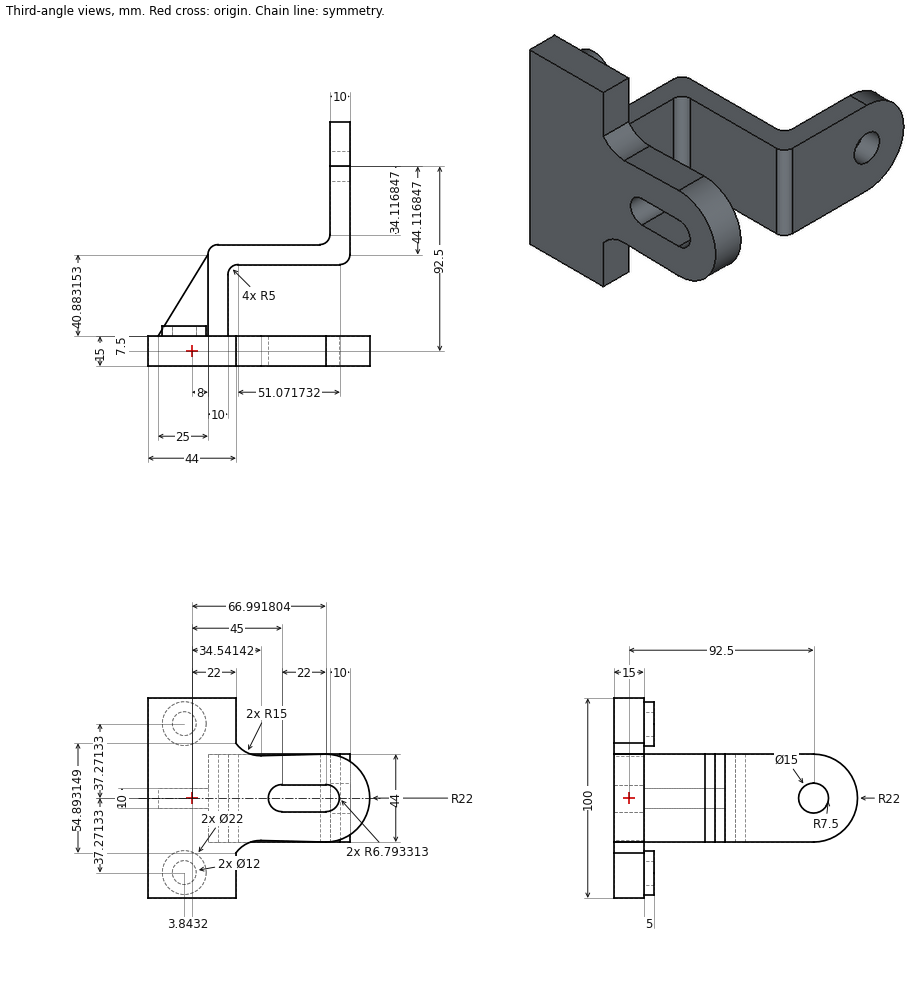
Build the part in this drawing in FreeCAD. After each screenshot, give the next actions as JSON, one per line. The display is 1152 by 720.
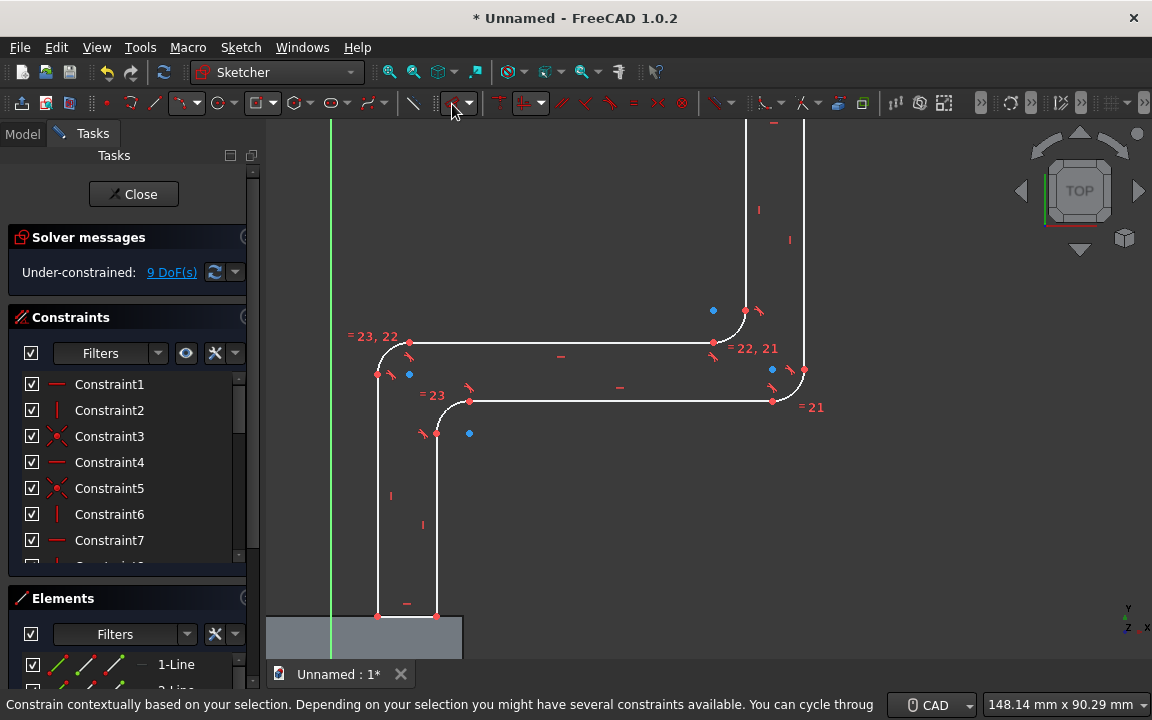
{"action": "scroll", "coordinate": [787, 398], "scroll_direction": "up", "scroll_amount": 2}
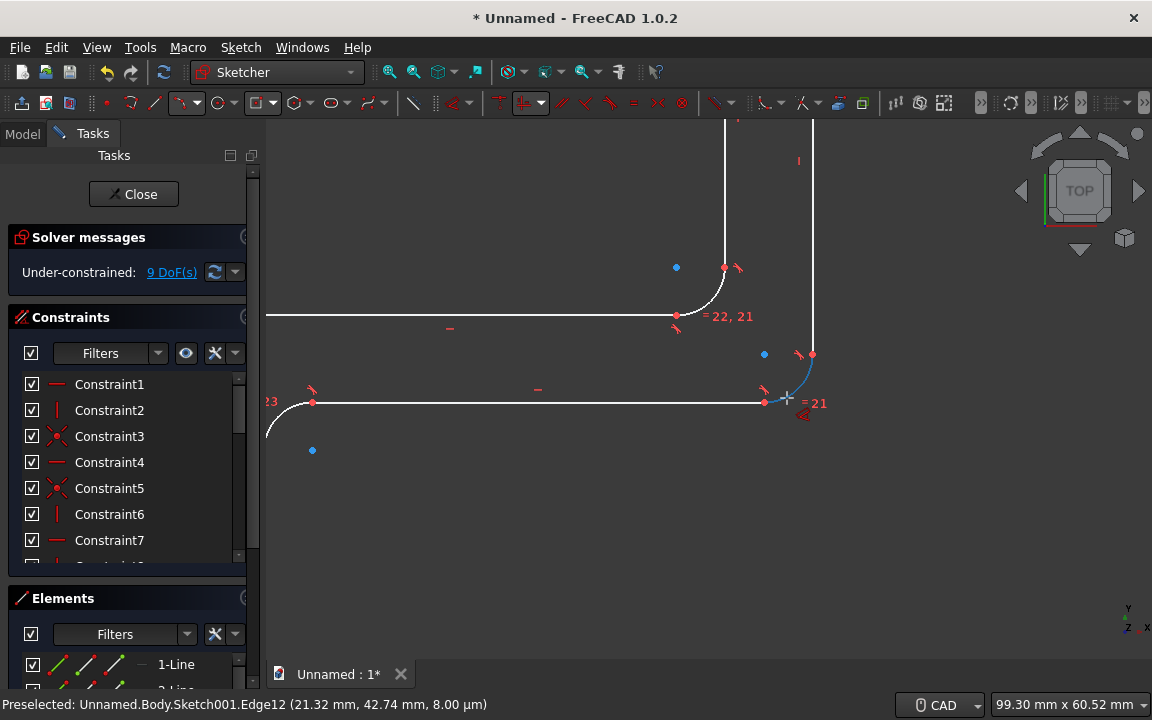
{"action": "left_click", "coordinate": [786, 397]}
{"action": "left_click", "coordinate": [800, 426]}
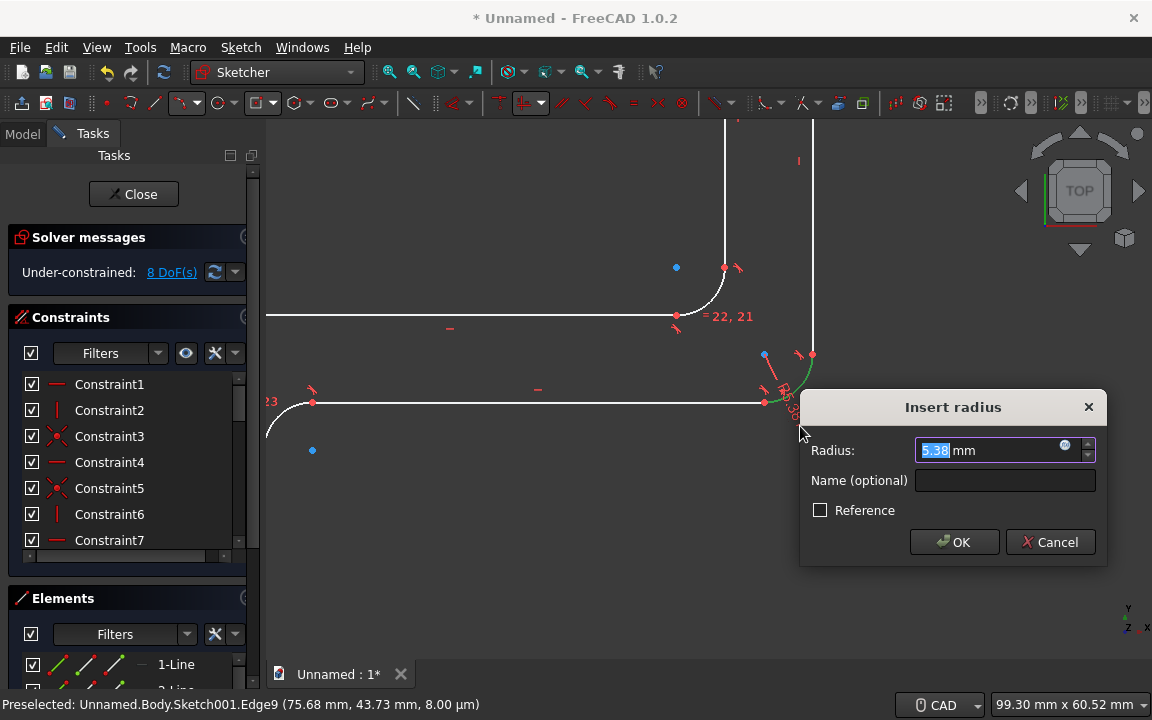
{"action": "type", "text": "5"}
{"action": "key", "text": "Return"}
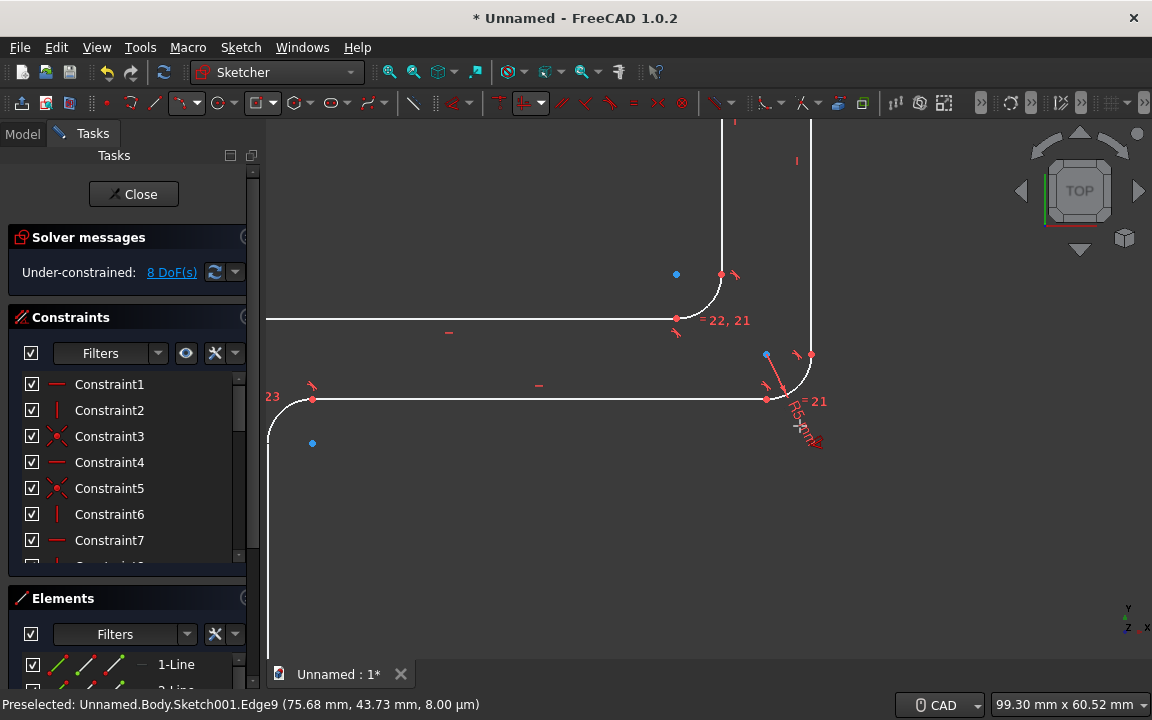
{"action": "scroll", "coordinate": [788, 399], "scroll_direction": "down", "scroll_amount": 4}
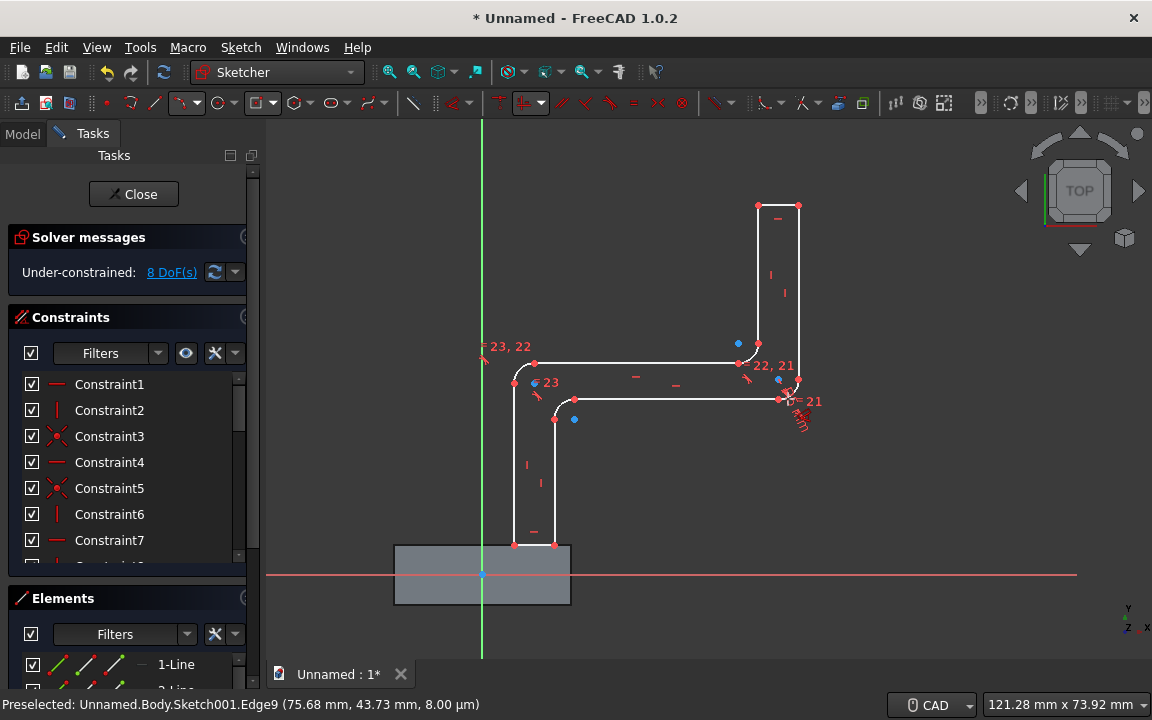
{"action": "left_click", "coordinate": [787, 205]}
{"action": "left_click", "coordinate": [779, 171]}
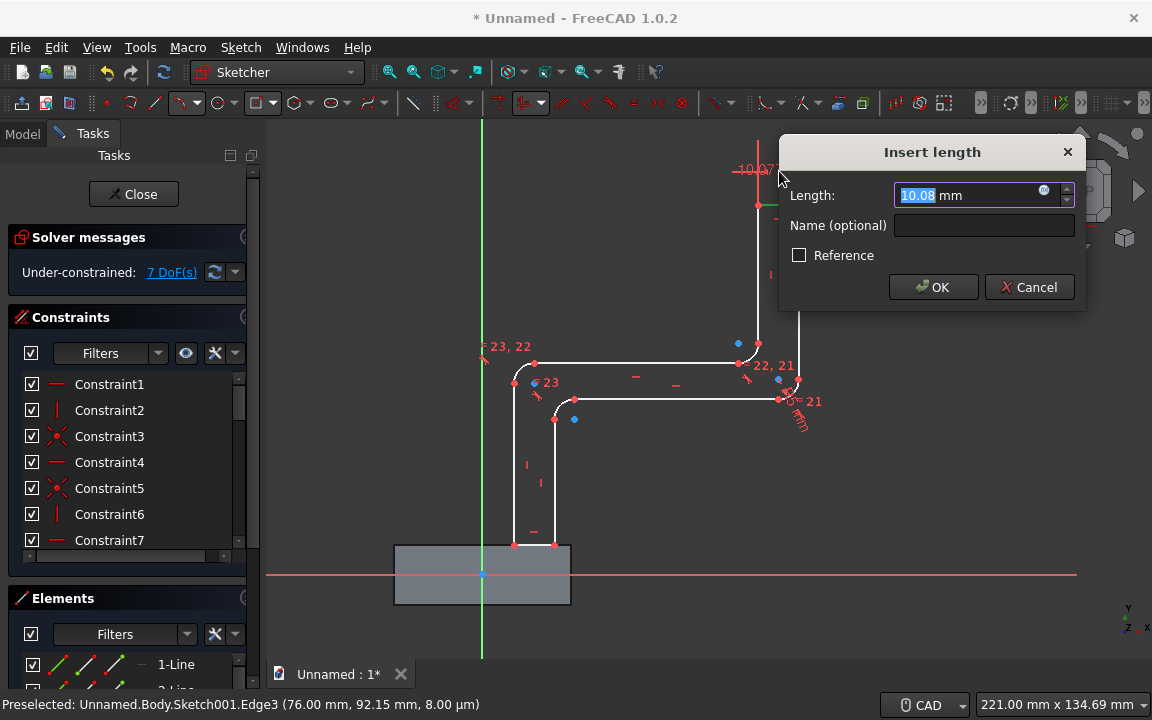
{"action": "type", "text": "10"}
{"action": "key", "text": "Return"}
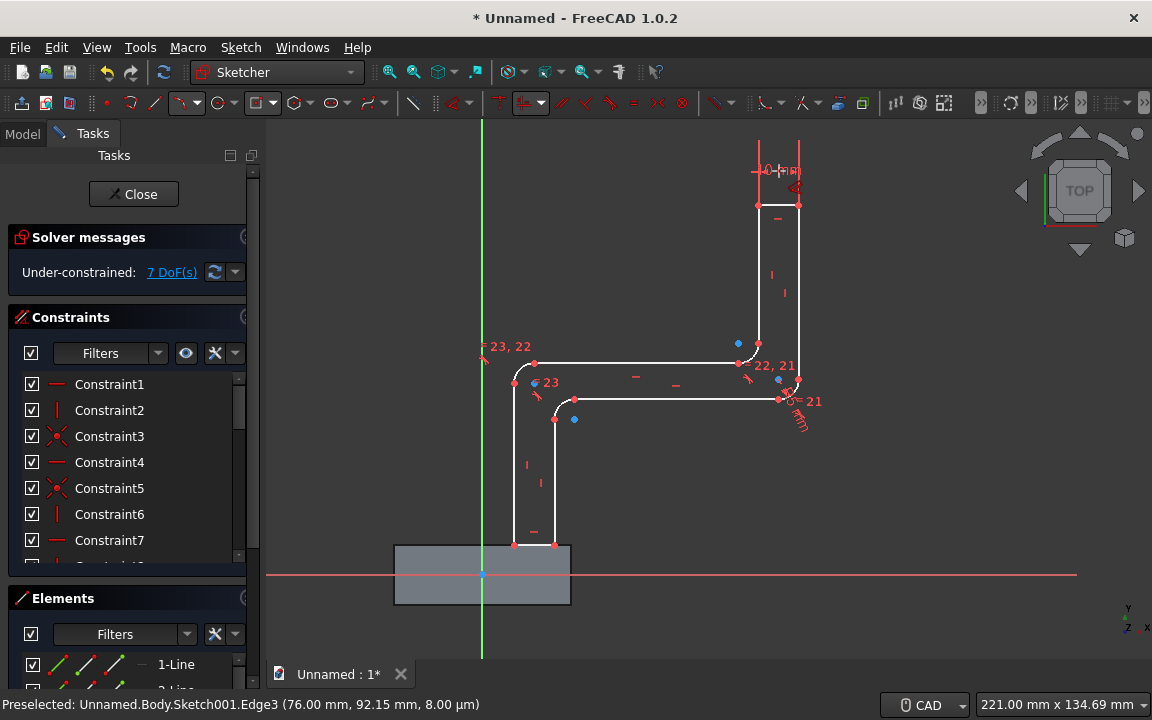
{"action": "left_click", "coordinate": [526, 545]}
{"action": "left_click", "coordinate": [534, 511]}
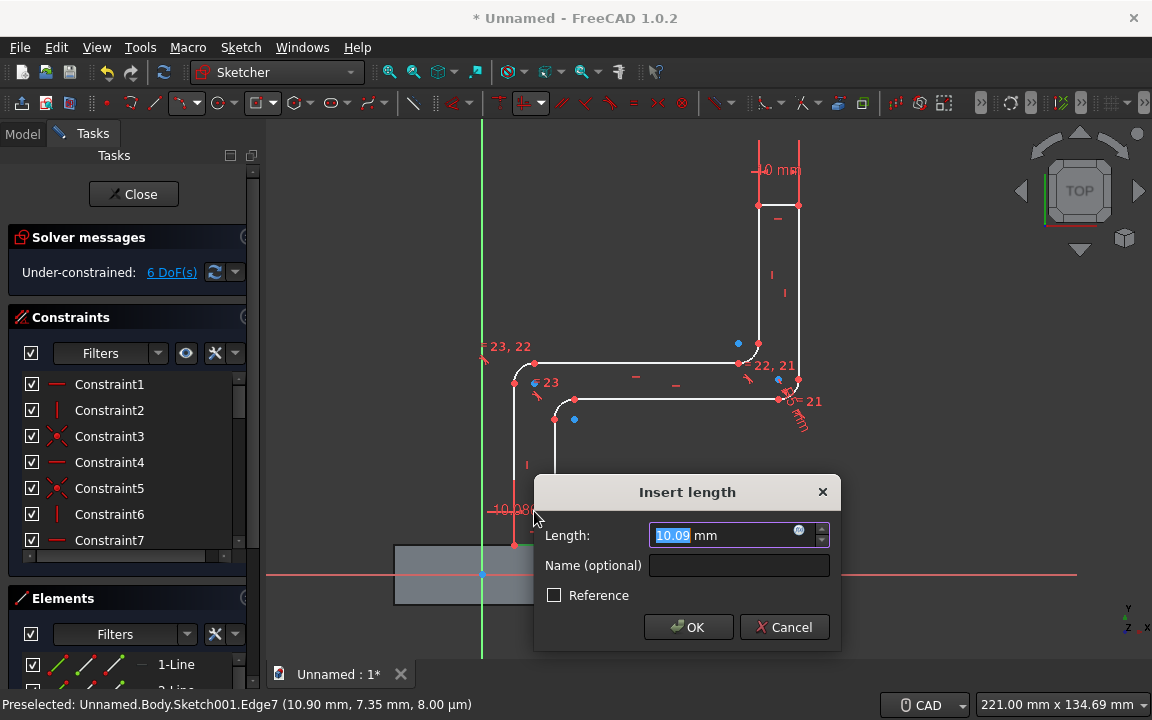
{"action": "type", "text": "10"}
{"action": "key", "text": "Return"}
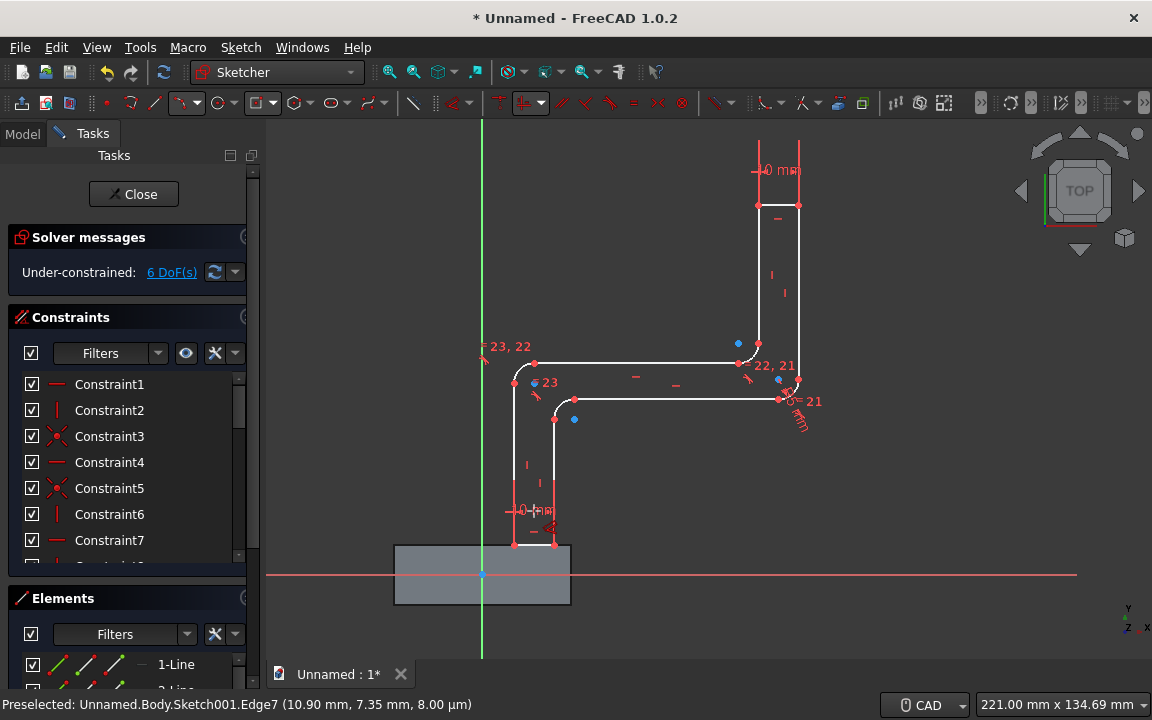
{"action": "scroll", "coordinate": [514, 383], "scroll_direction": "up", "scroll_amount": 2}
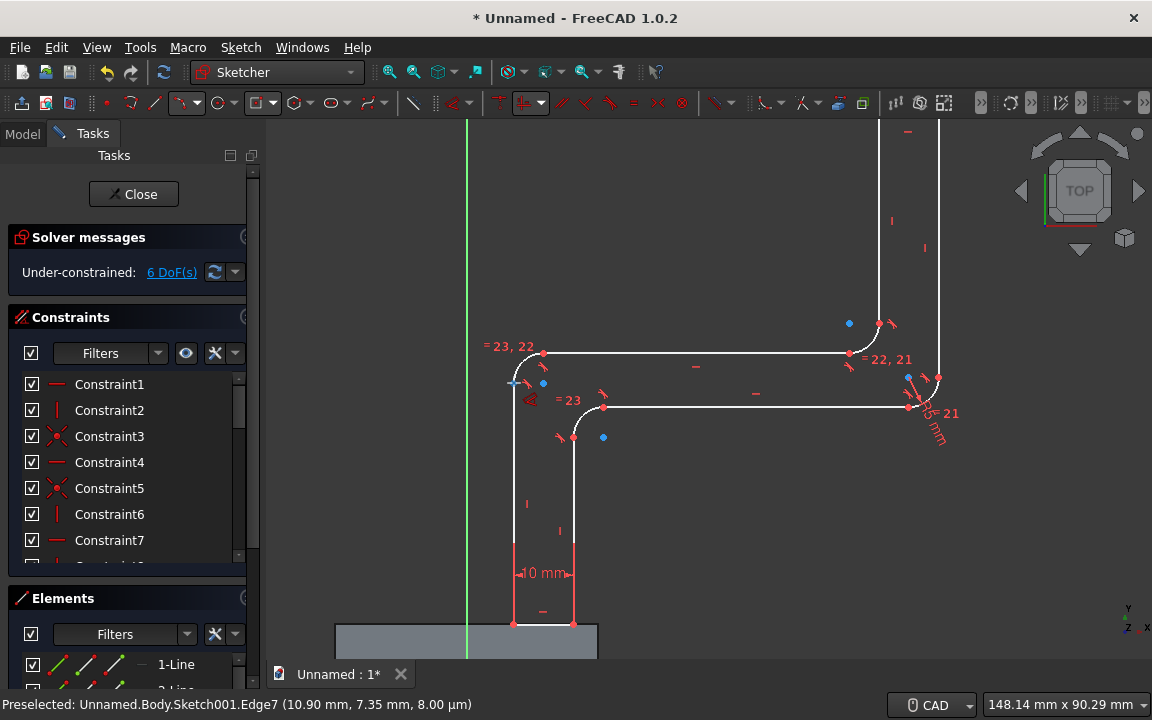
{"action": "left_click", "coordinate": [514, 383]}
{"action": "left_click", "coordinate": [490, 349]}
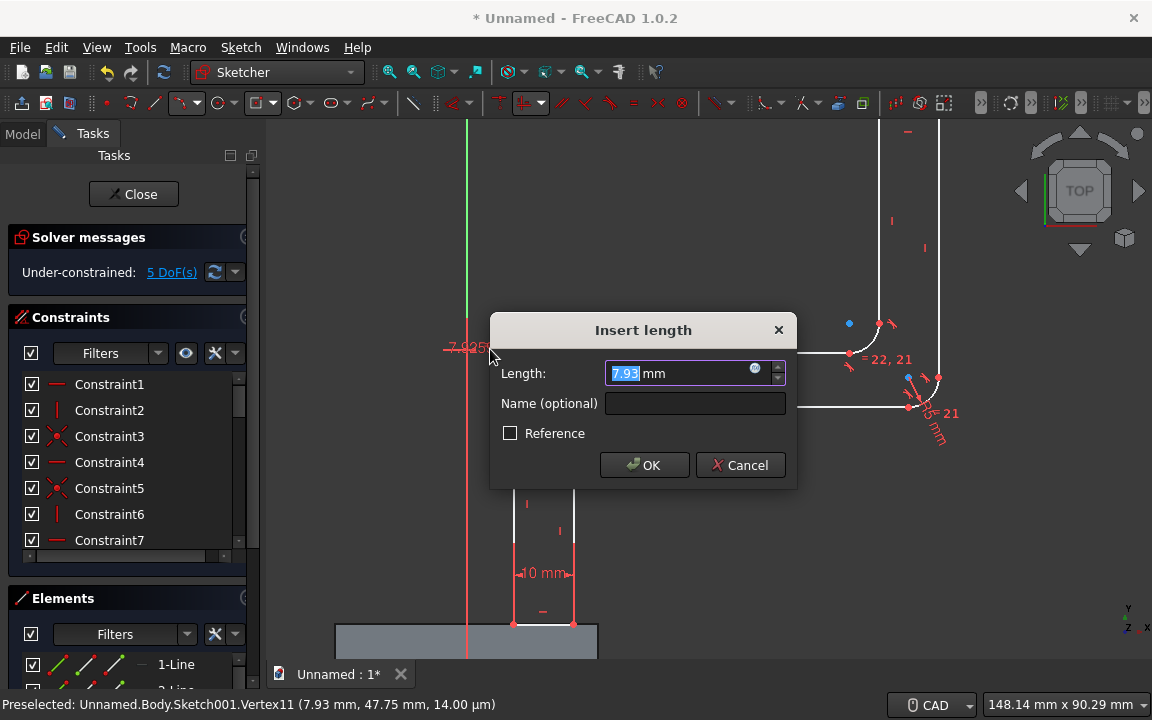
{"action": "type", "text": "8"}
{"action": "key", "text": "Return"}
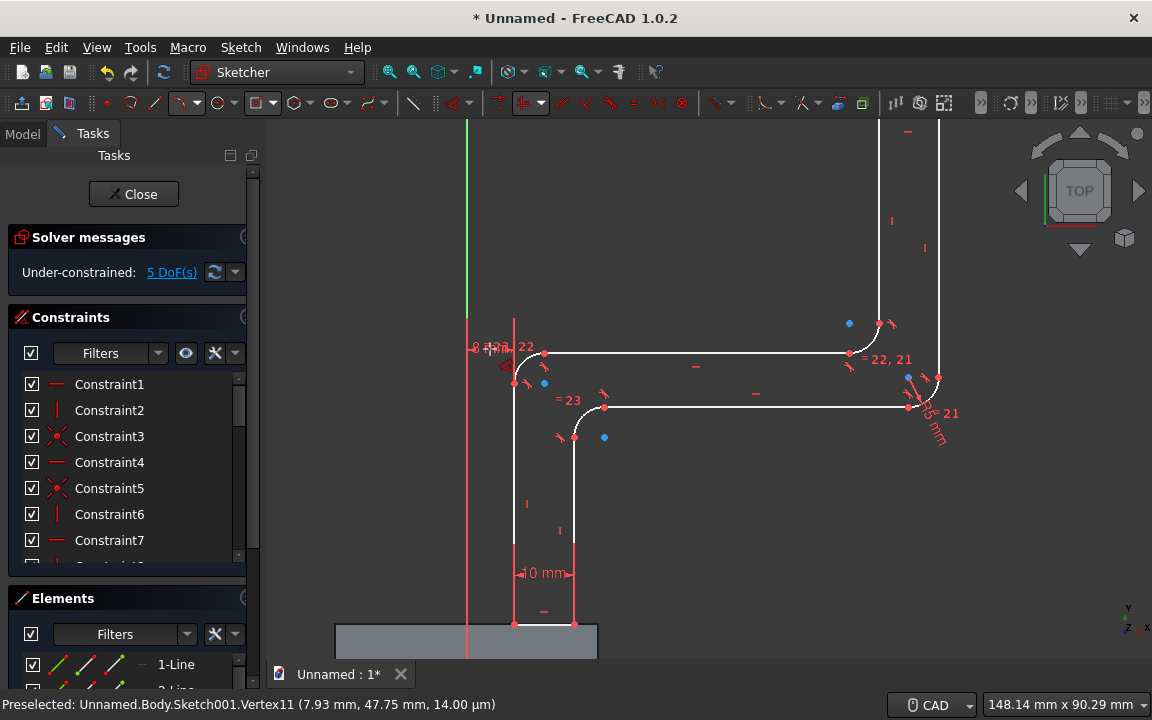
{"action": "left_click", "coordinate": [514, 625]}
{"action": "left_click", "coordinate": [433, 628]}